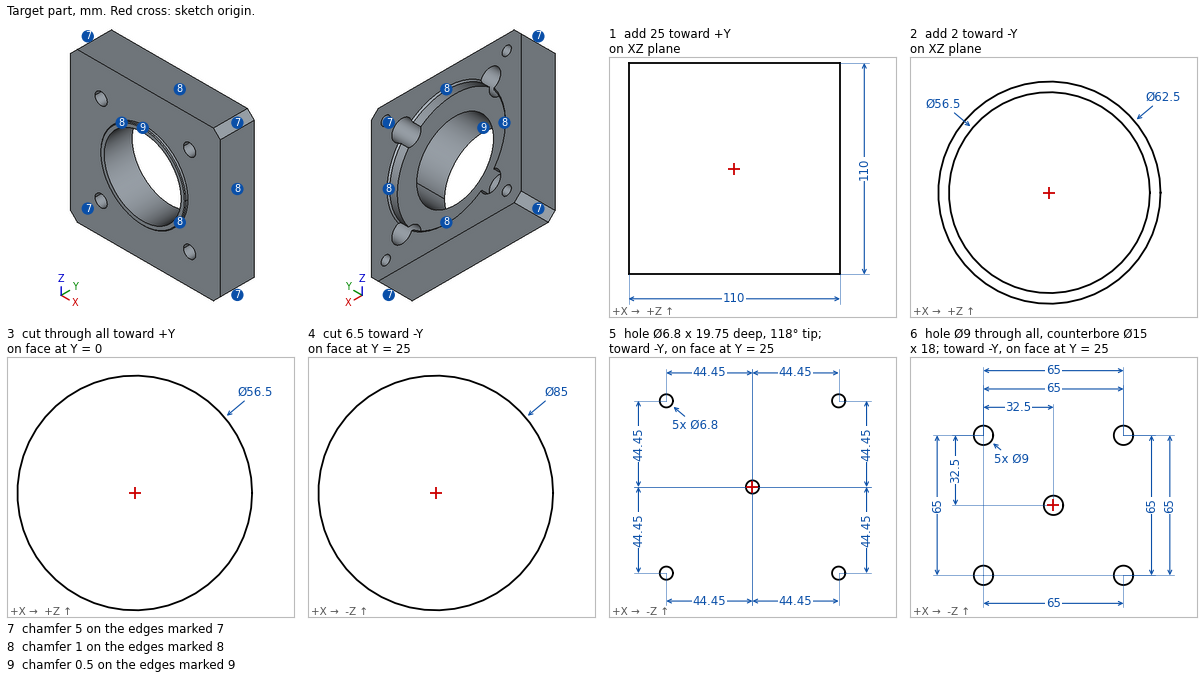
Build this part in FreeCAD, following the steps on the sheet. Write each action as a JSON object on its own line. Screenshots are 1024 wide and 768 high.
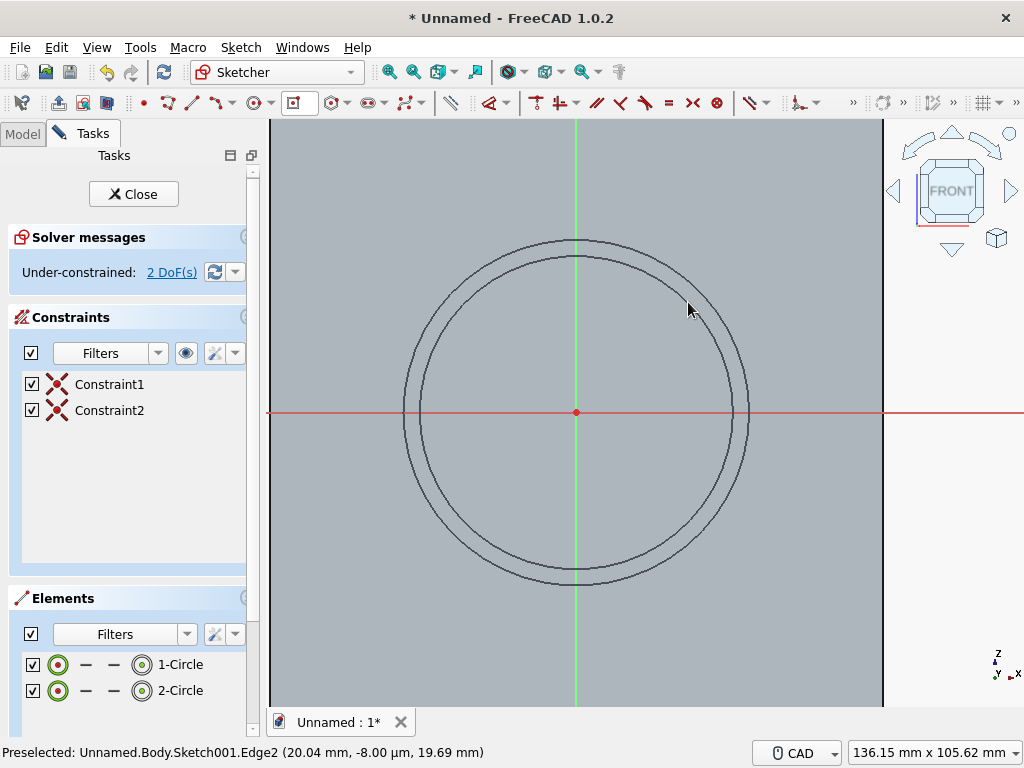
{"action": "left_click", "coordinate": [490, 104]}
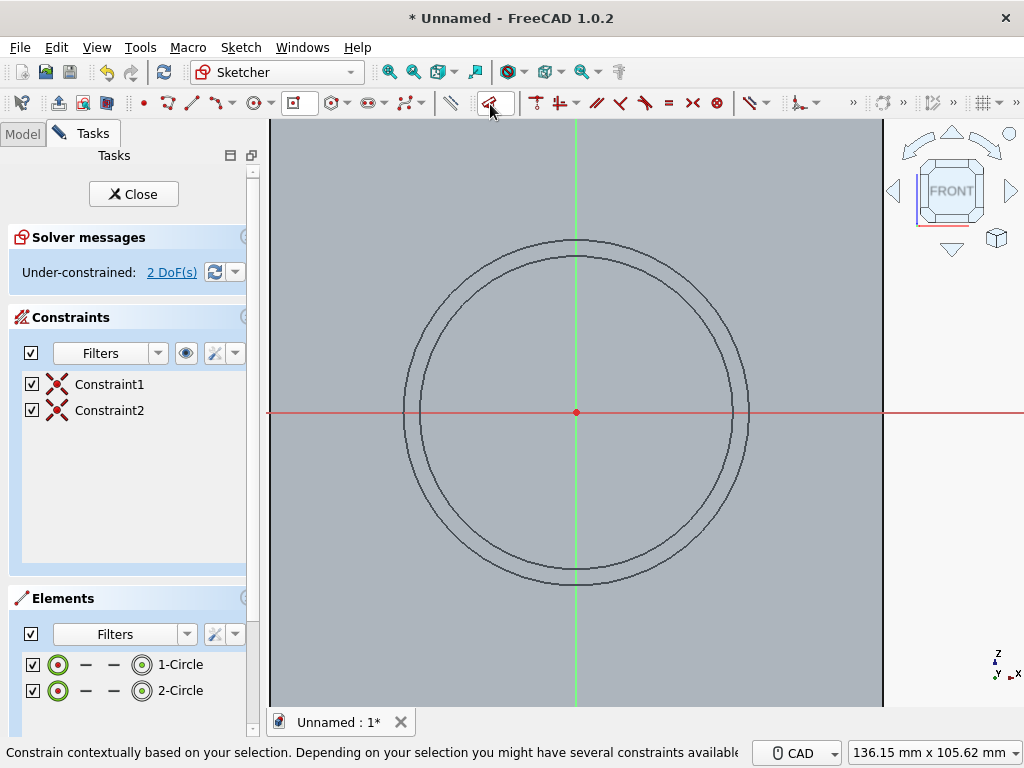
{"action": "left_click", "coordinate": [698, 290]}
{"action": "left_click", "coordinate": [721, 267]}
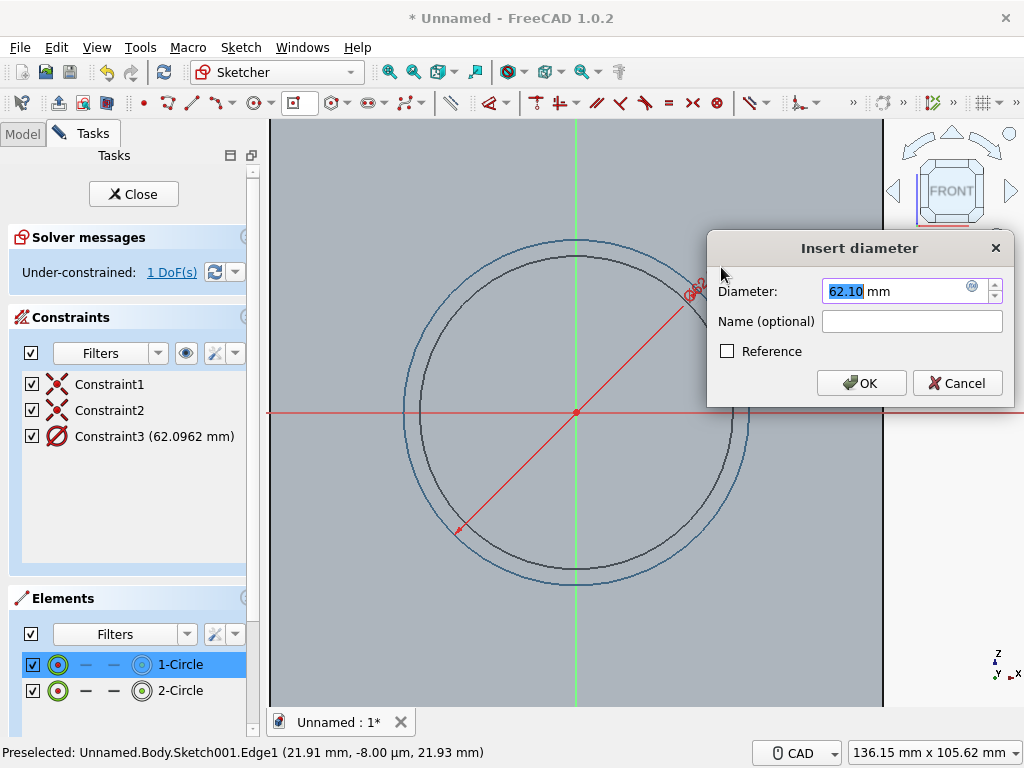
{"action": "type", "text": "62.5"}
{"action": "key", "text": "Return"}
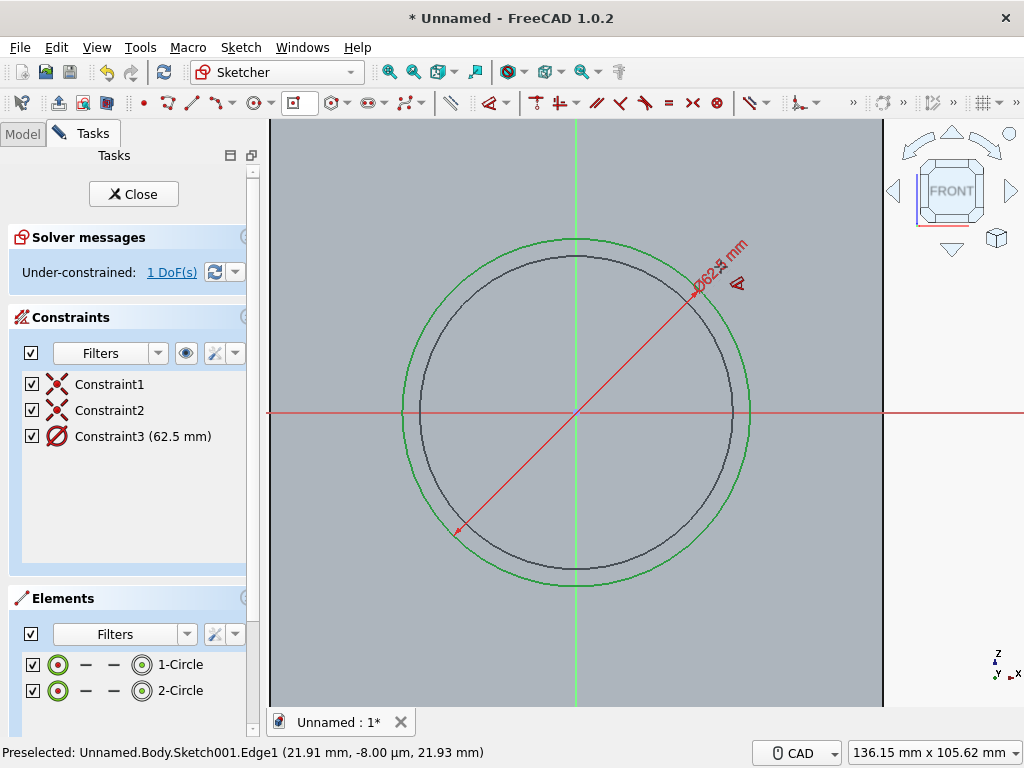
{"action": "left_click", "coordinate": [687, 302]}
{"action": "left_click", "coordinate": [757, 360]}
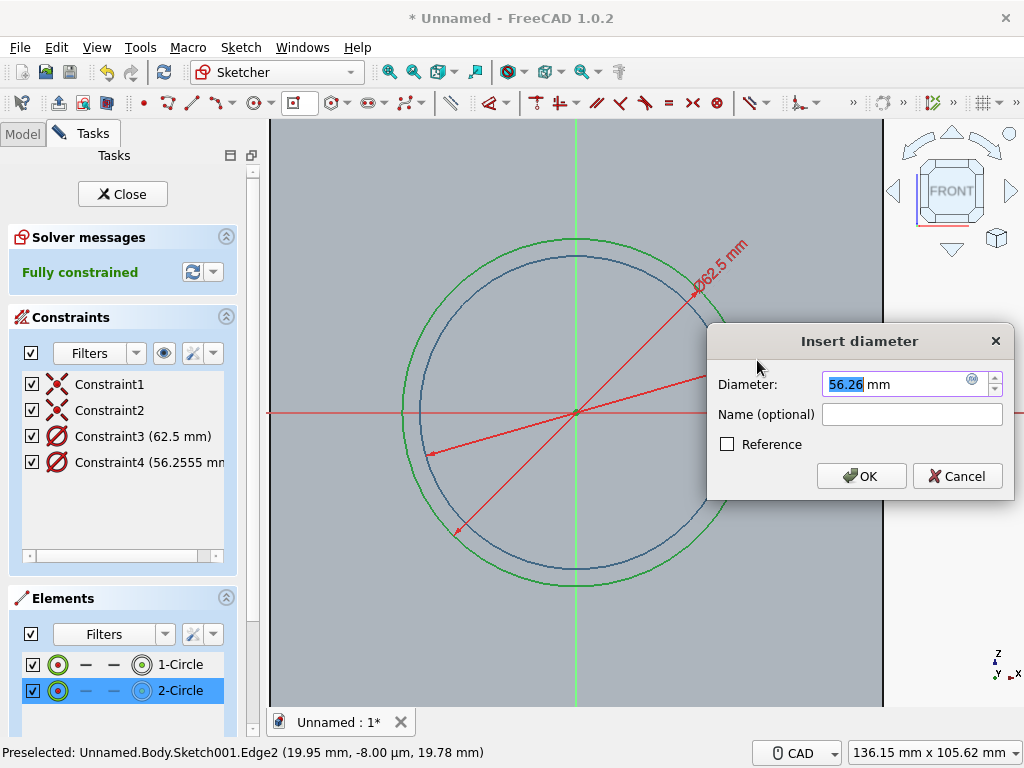
{"action": "type", "text": "56.5"}
{"action": "key", "text": "Return"}
{"action": "key", "text": "Escape"}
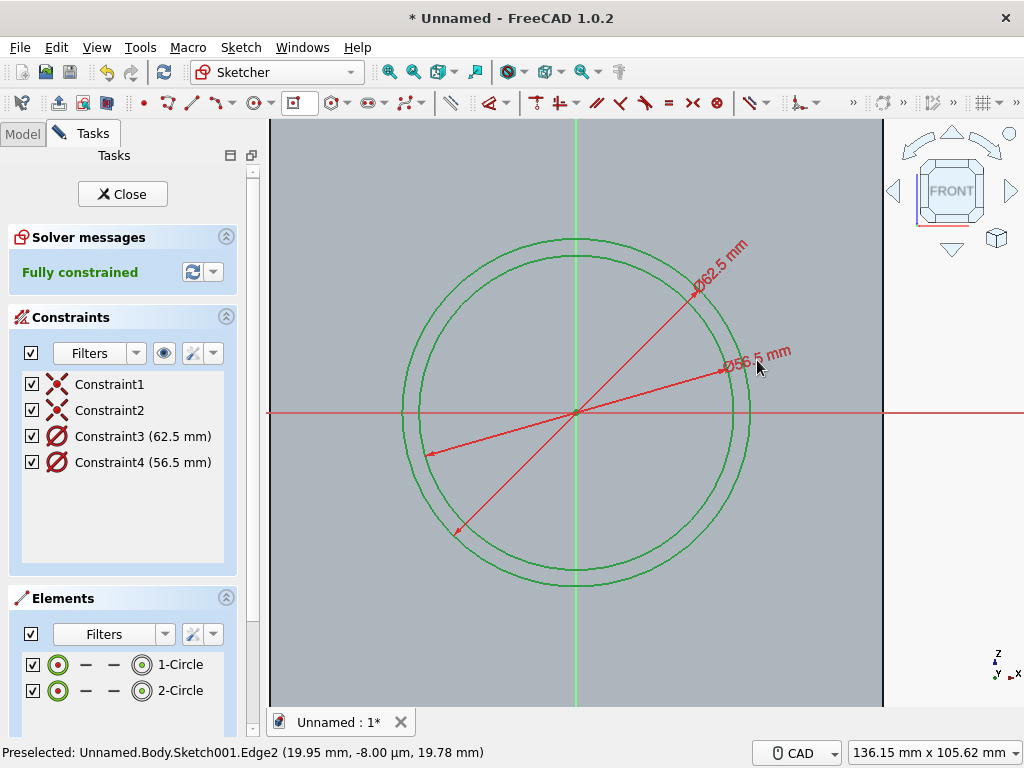
{"action": "left_click", "coordinate": [123, 194]}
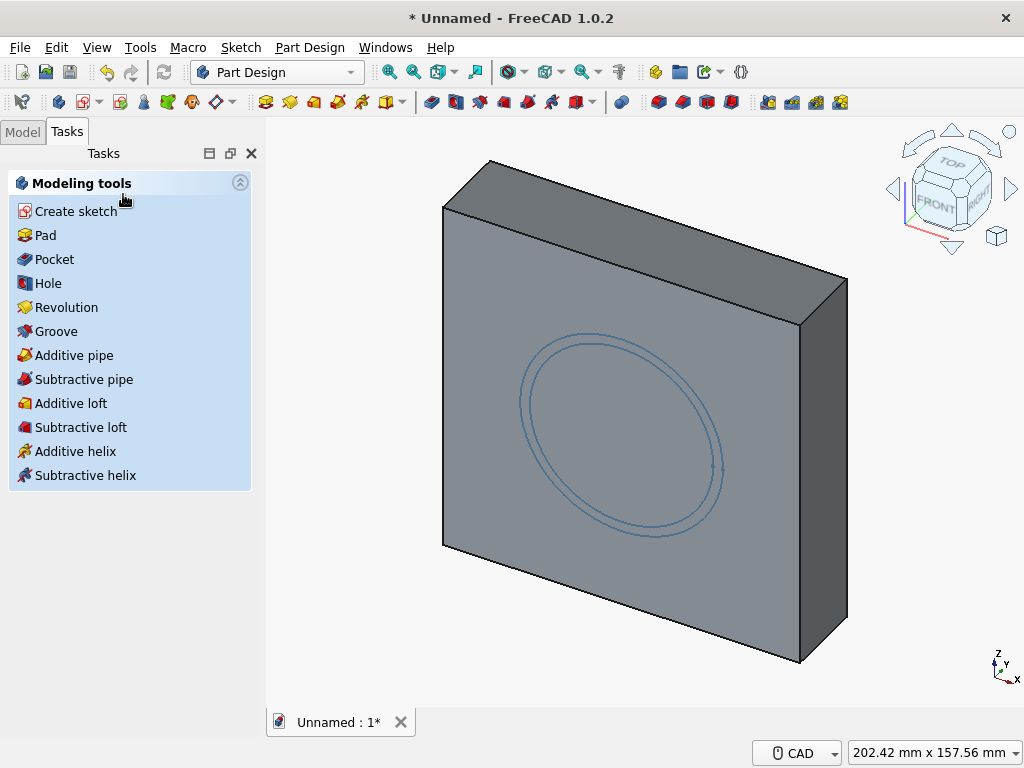
{"action": "left_click", "coordinate": [266, 102]}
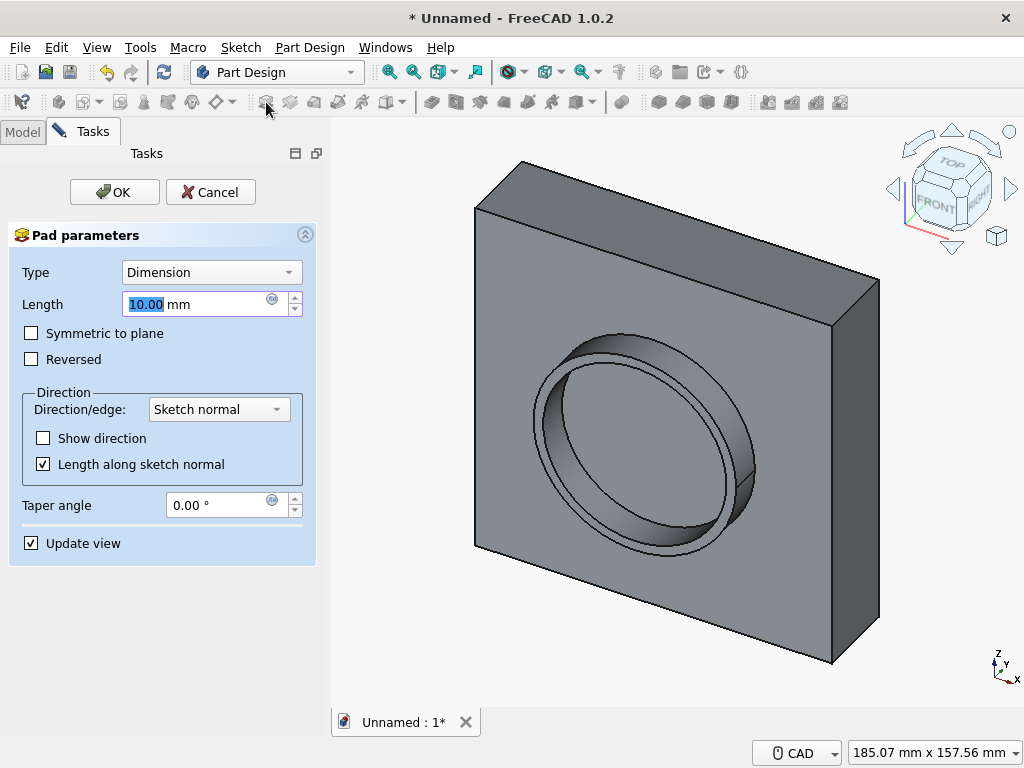
{"action": "type", "text": "2"}
{"action": "key", "text": "Tab"}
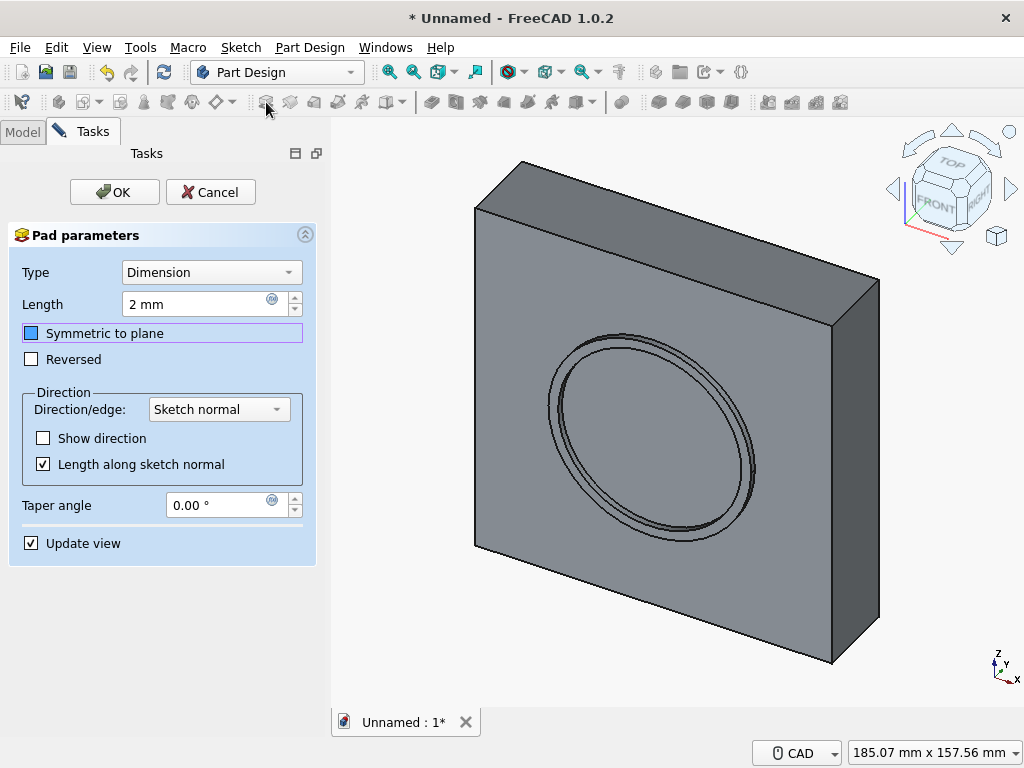
{"action": "left_click", "coordinate": [115, 192]}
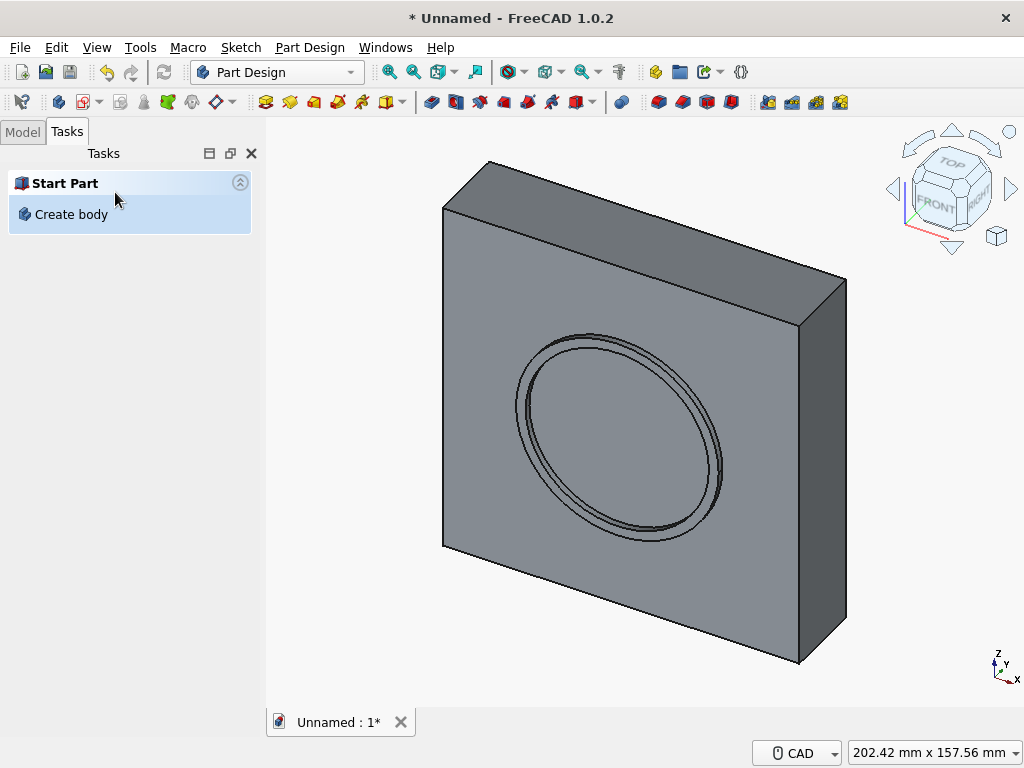
{"action": "left_click", "coordinate": [723, 372]}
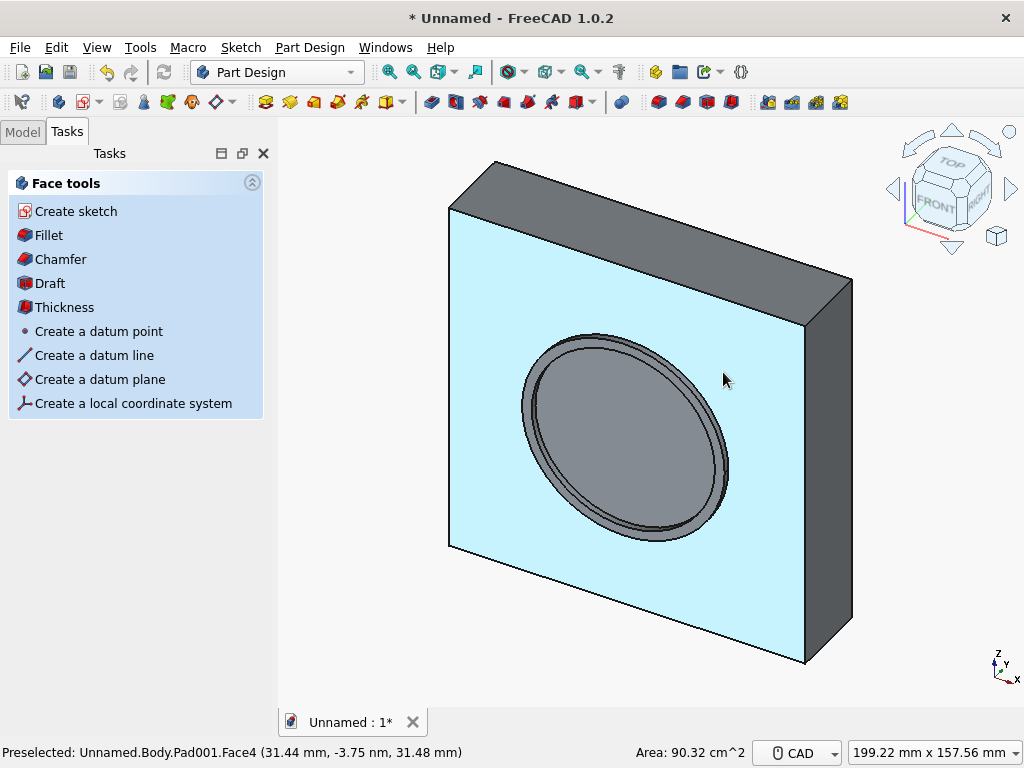
{"action": "left_click", "coordinate": [84, 102]}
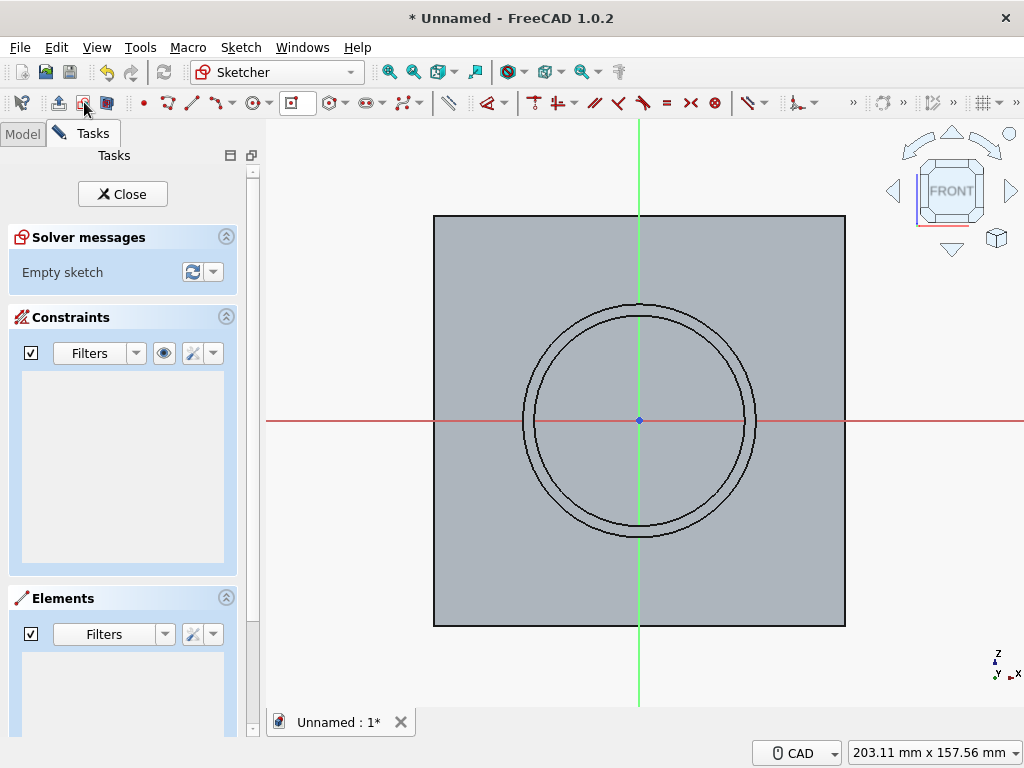
{"action": "scroll", "coordinate": [716, 430], "scroll_direction": "up", "scroll_amount": 3}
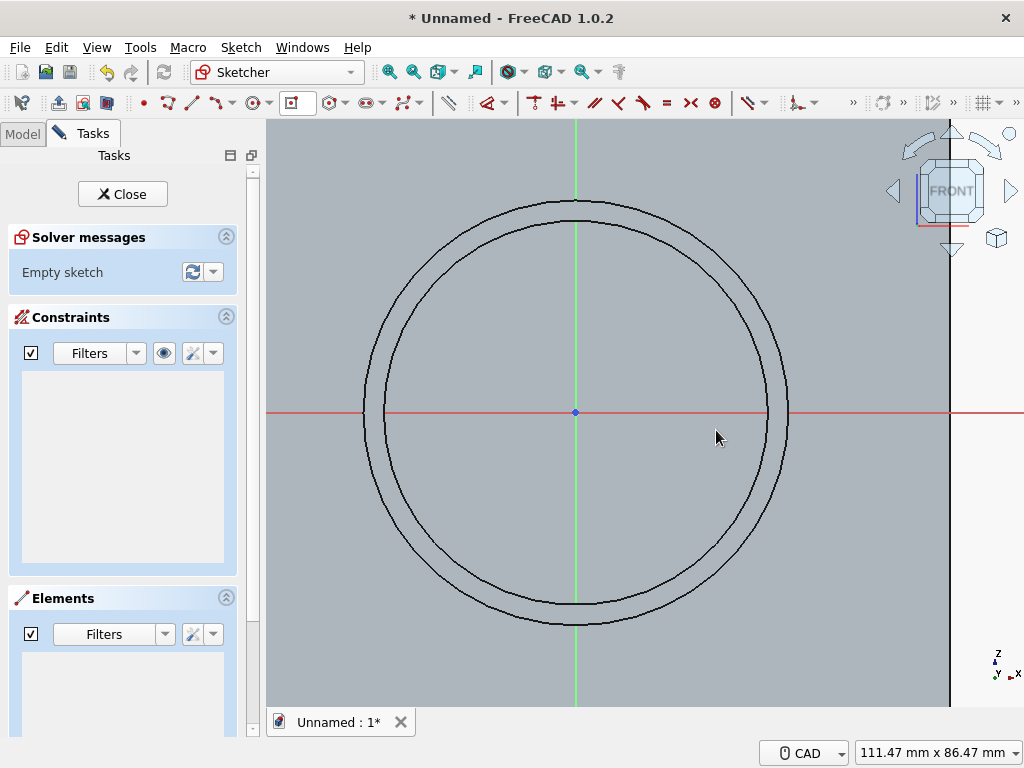
{"action": "left_click", "coordinate": [254, 104]}